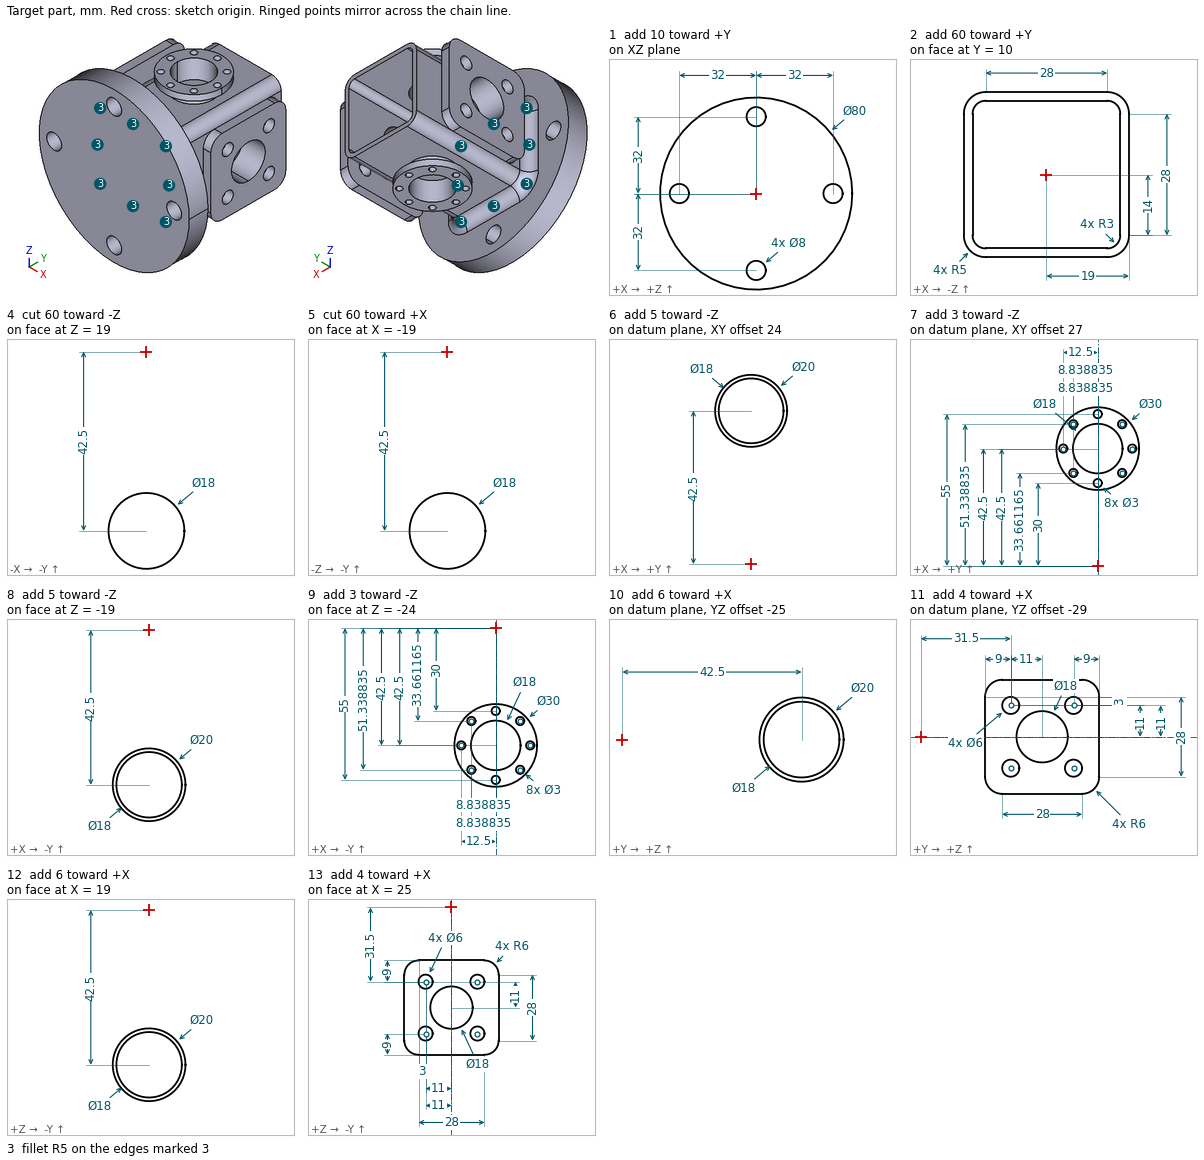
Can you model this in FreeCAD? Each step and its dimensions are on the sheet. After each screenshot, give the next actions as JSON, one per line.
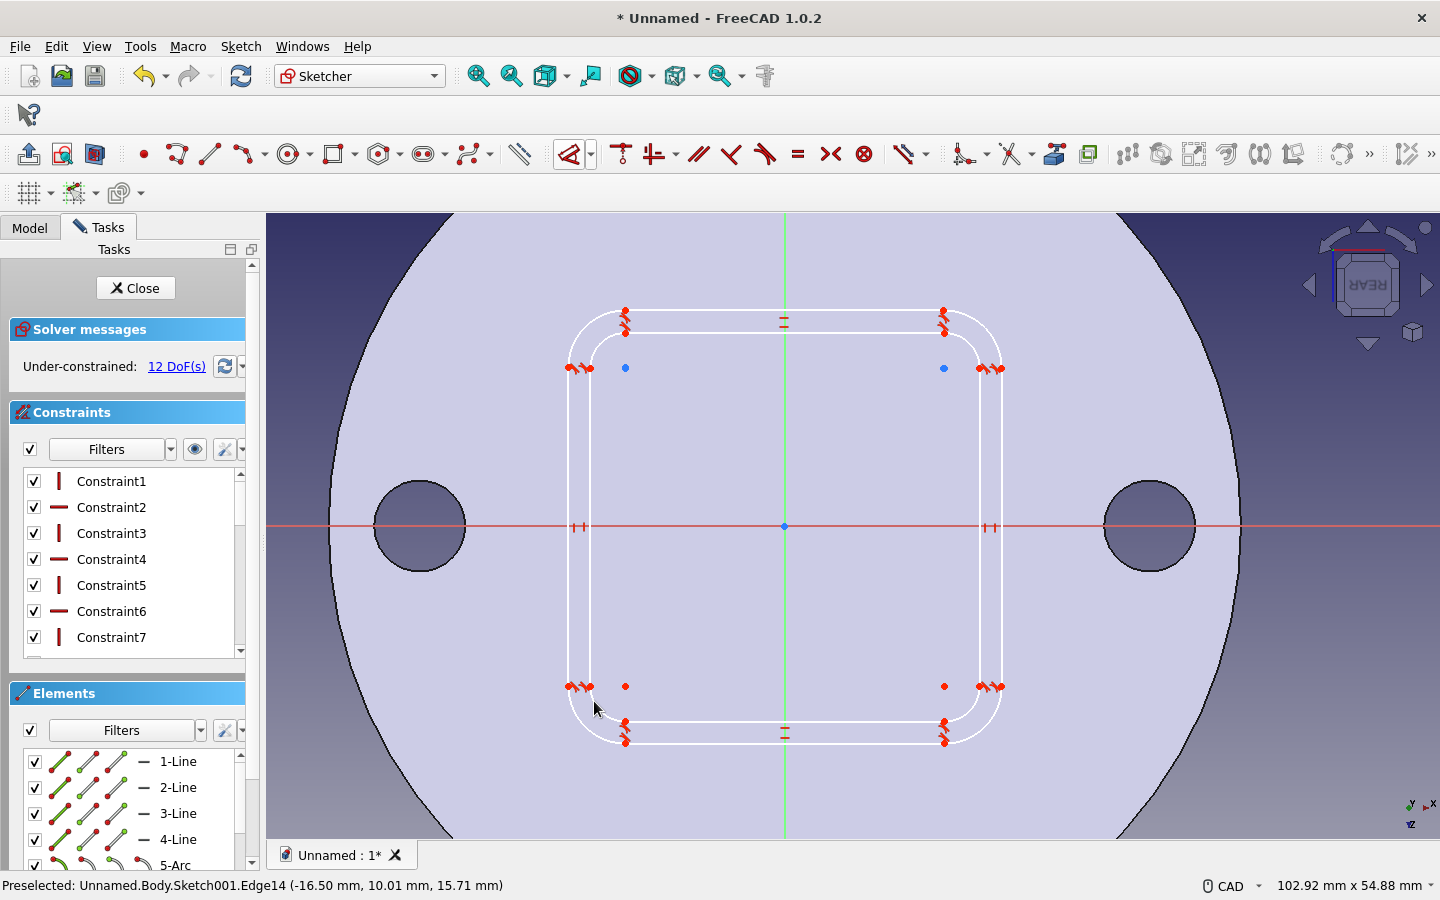
{"action": "left_click", "coordinate": [600, 317]}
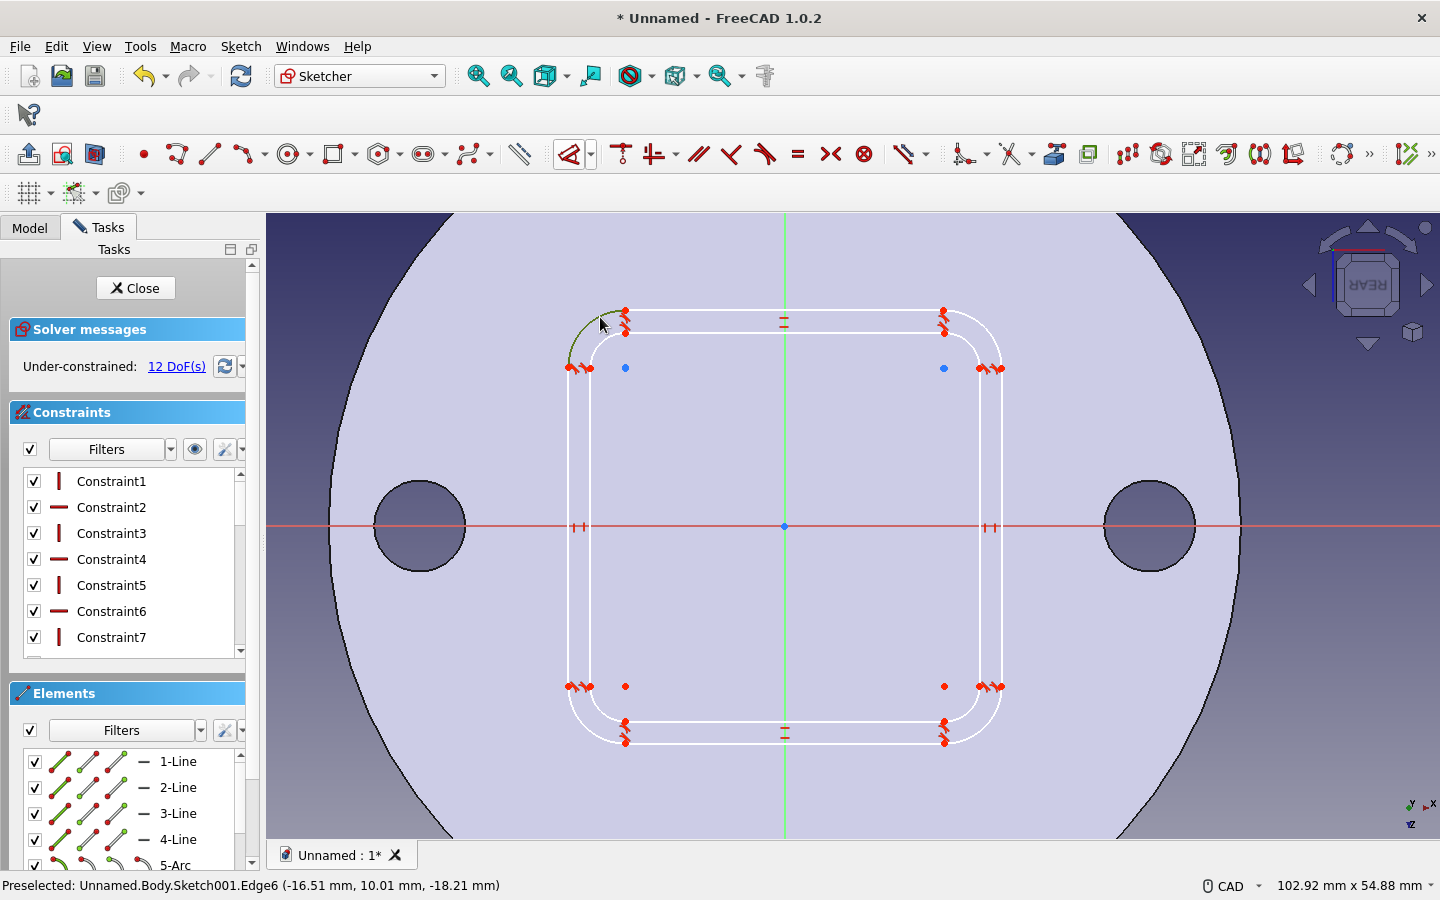
{"action": "left_click", "coordinate": [610, 337]}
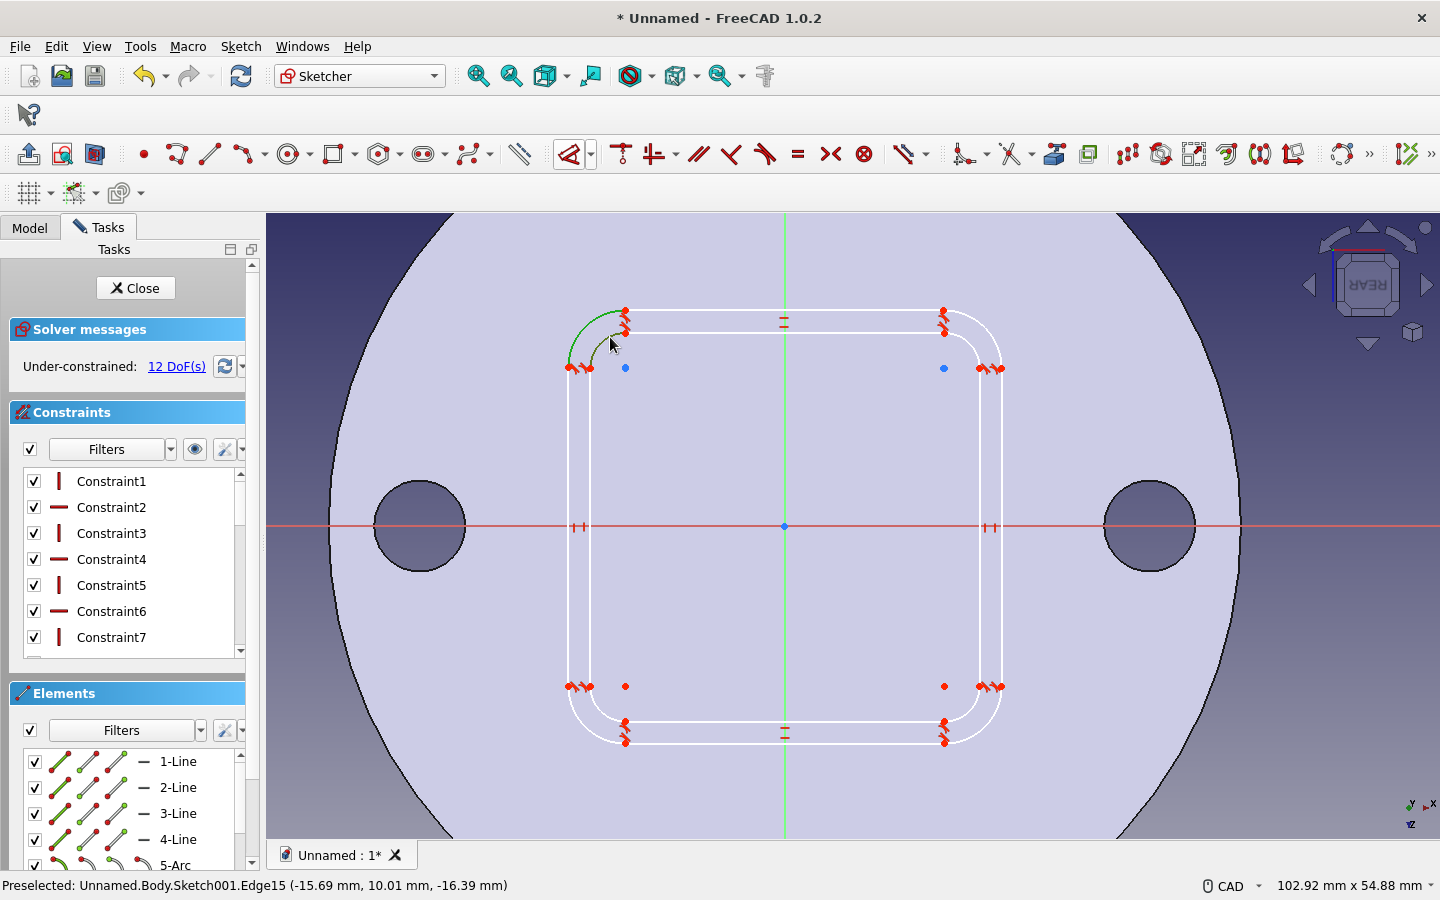
{"action": "key", "text": "c"}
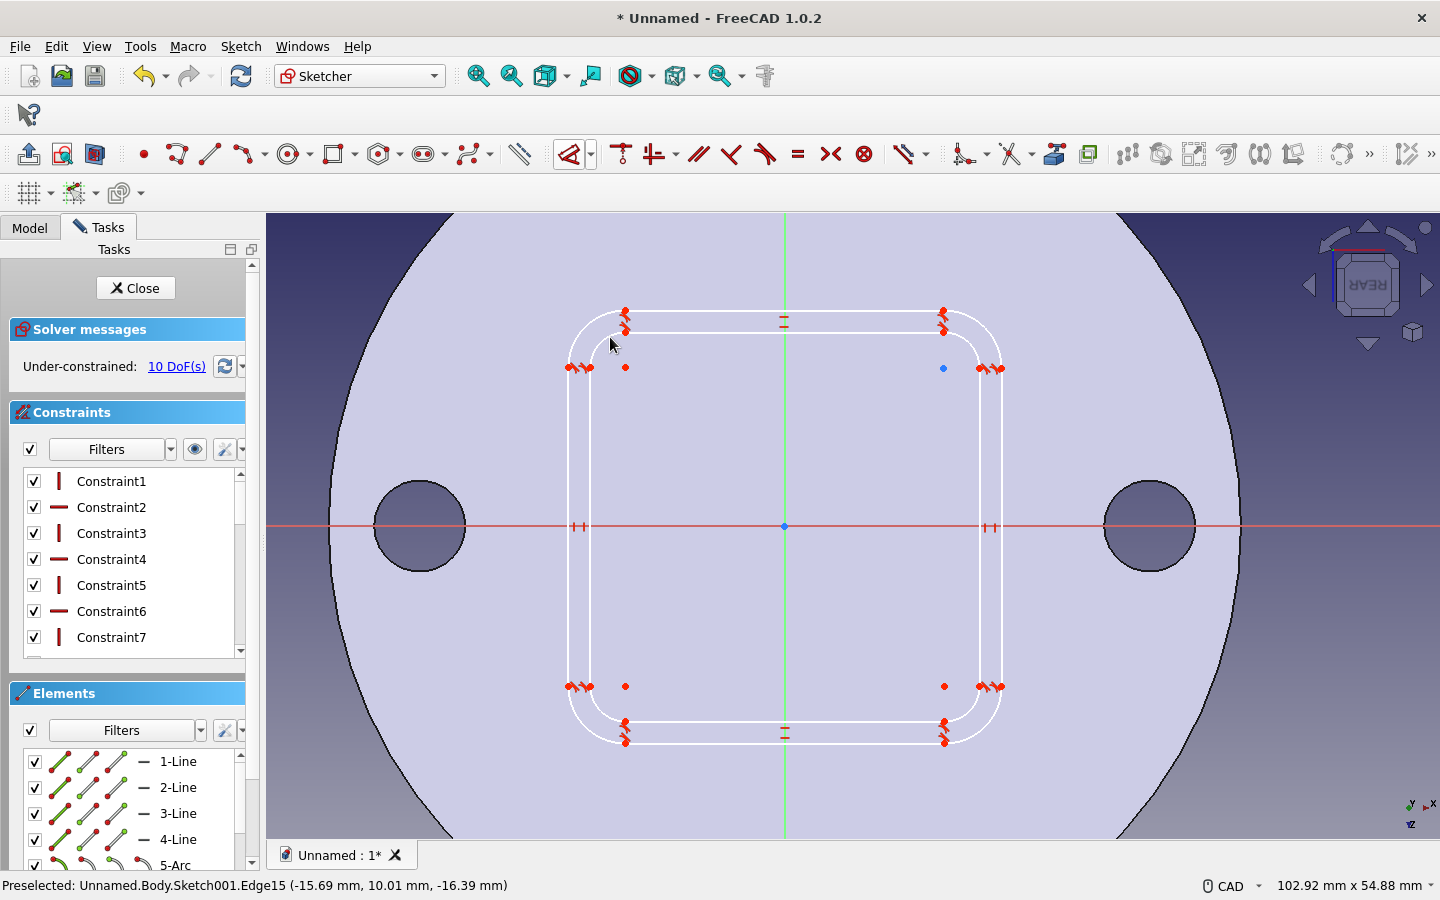
{"action": "left_click", "coordinate": [995, 342]}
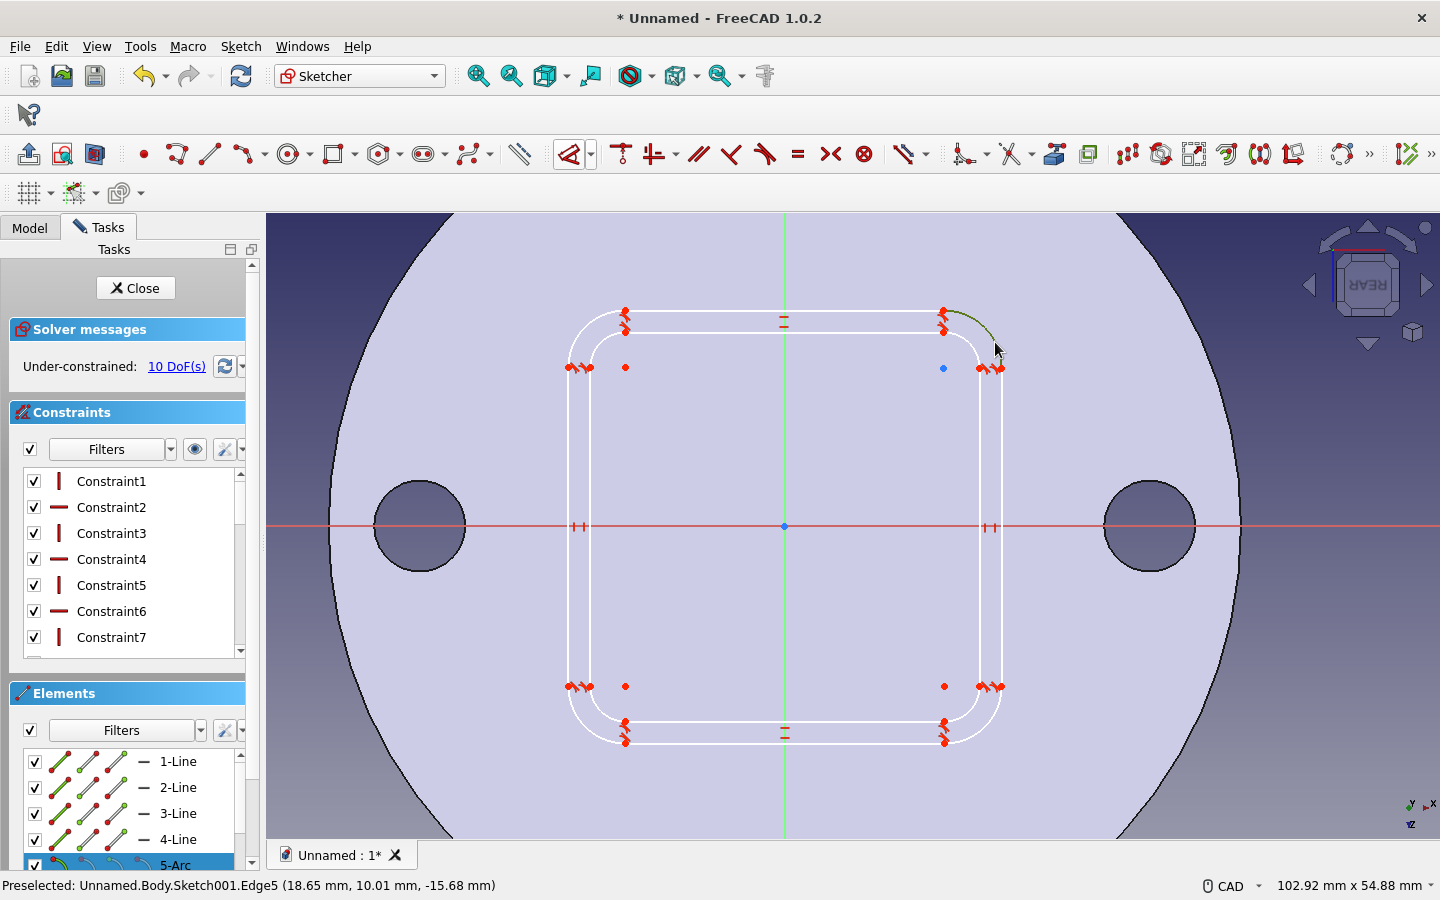
{"action": "left_click", "coordinate": [600, 317]}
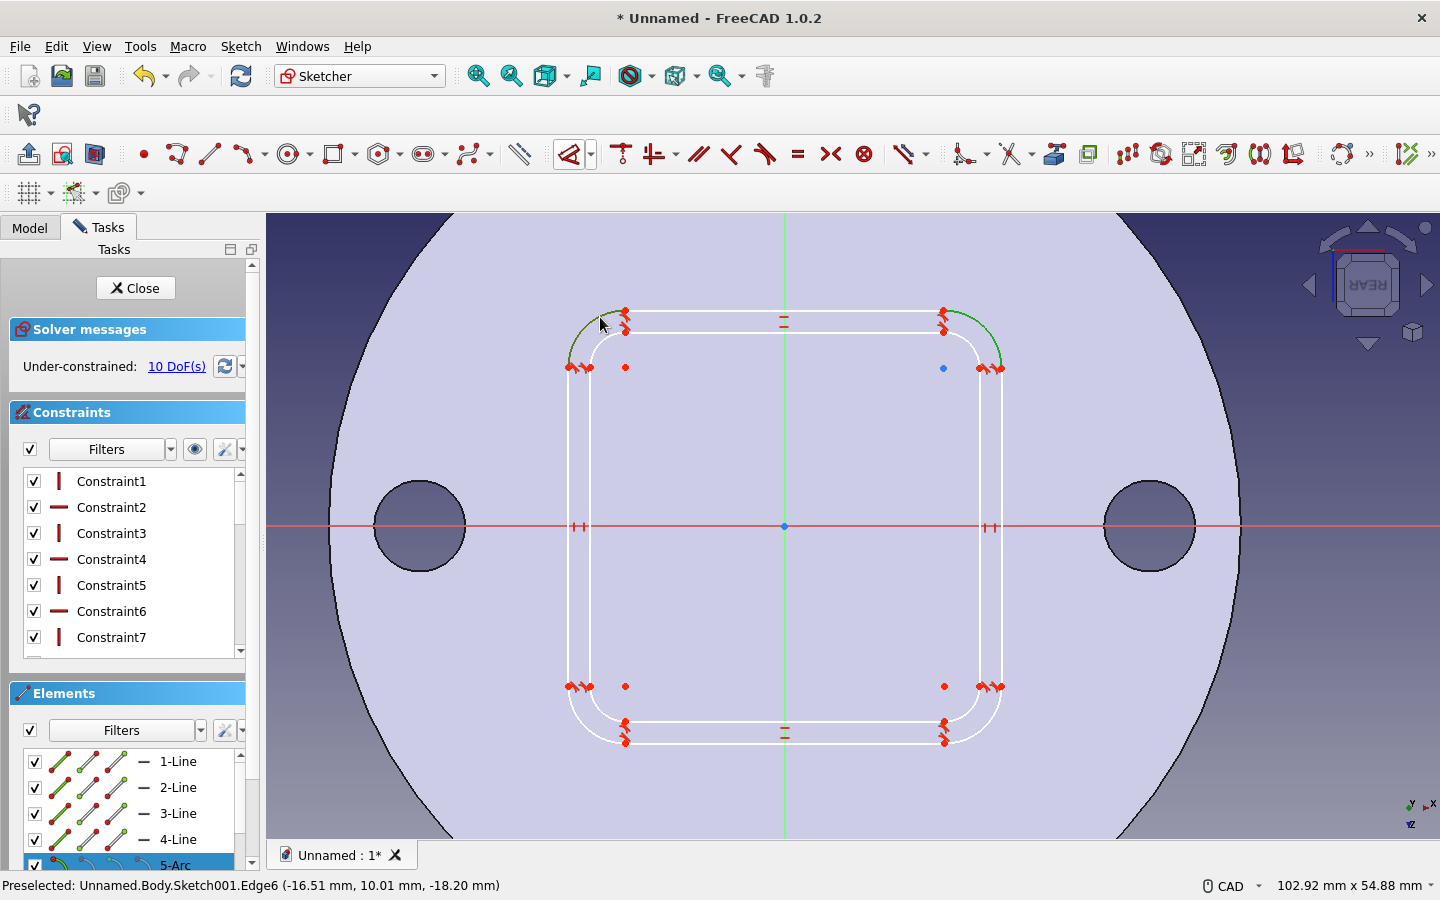
{"action": "left_click", "coordinate": [575, 712]}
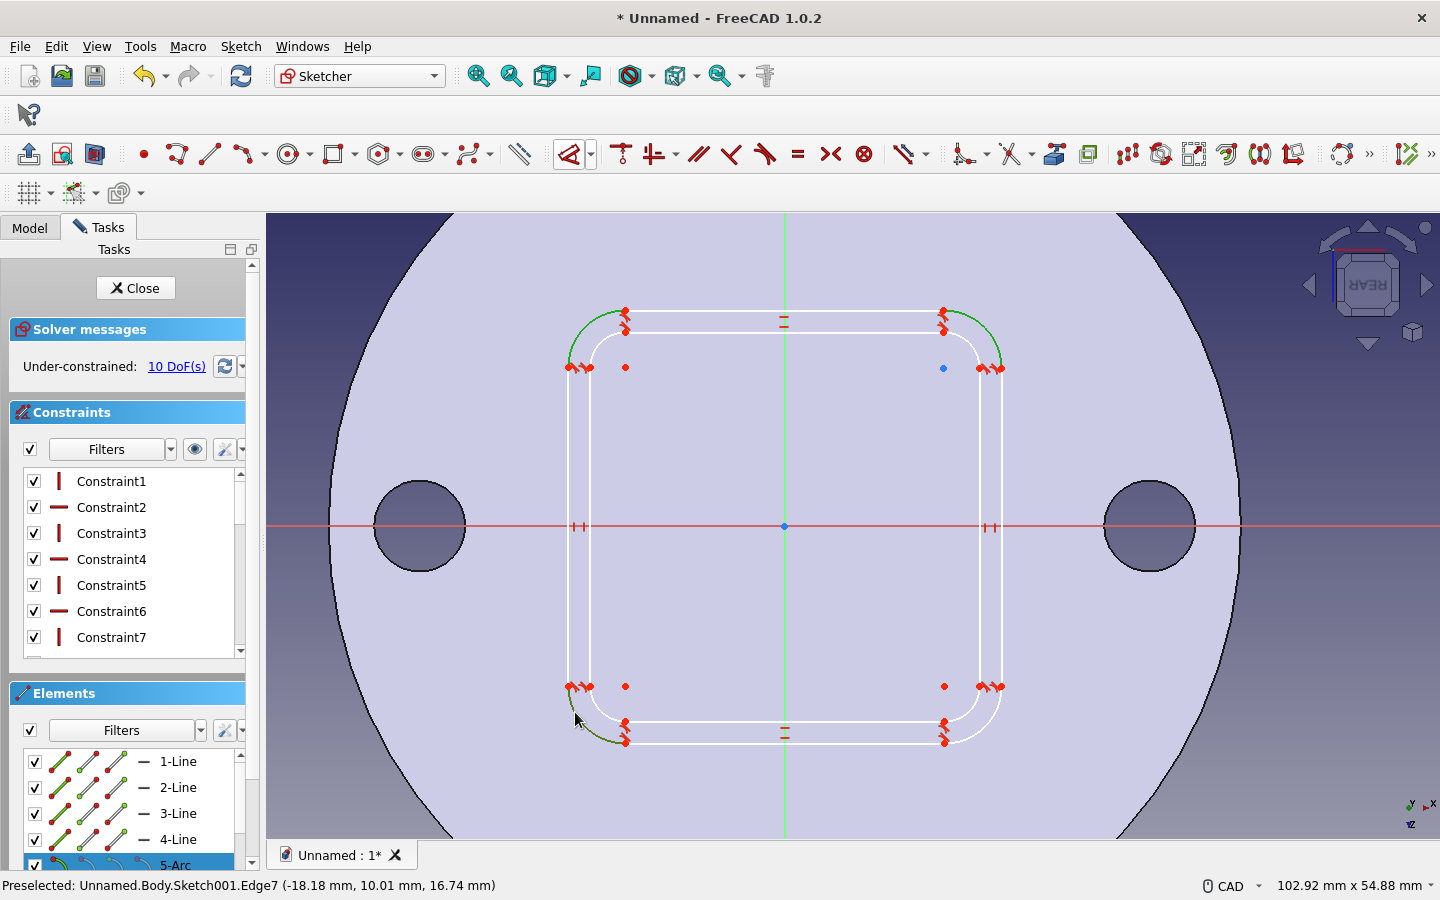
{"action": "left_click", "coordinate": [970, 737]}